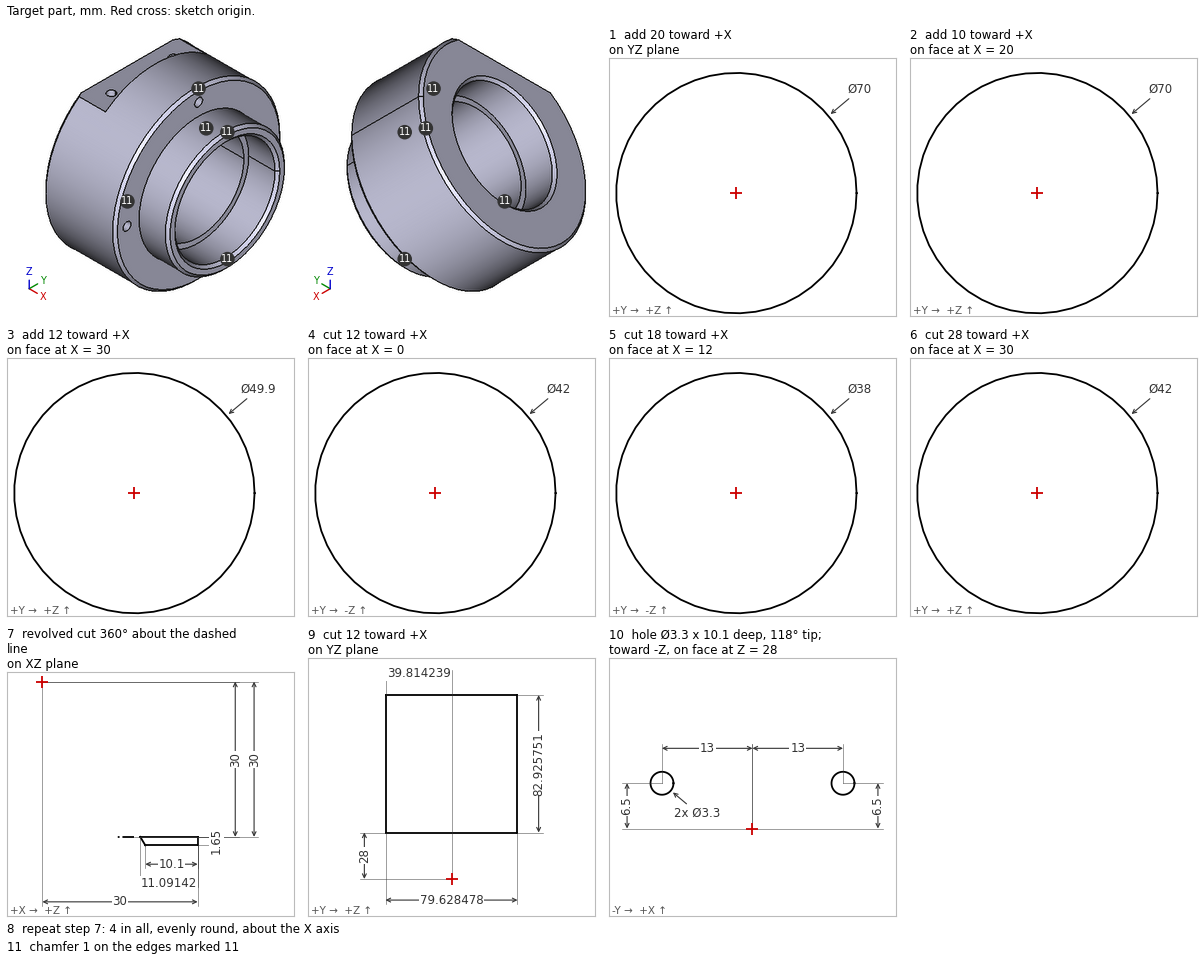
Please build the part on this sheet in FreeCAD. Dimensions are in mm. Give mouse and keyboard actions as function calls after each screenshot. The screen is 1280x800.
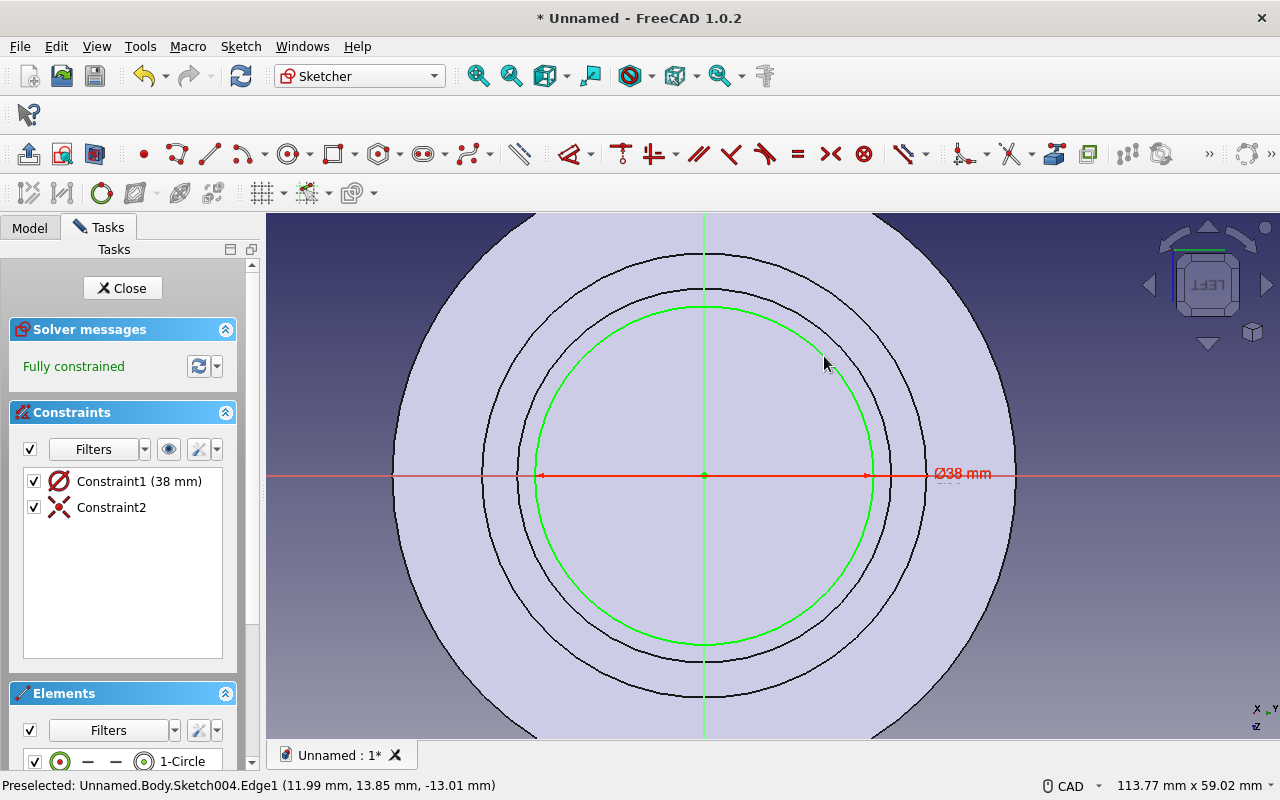
click(123, 288)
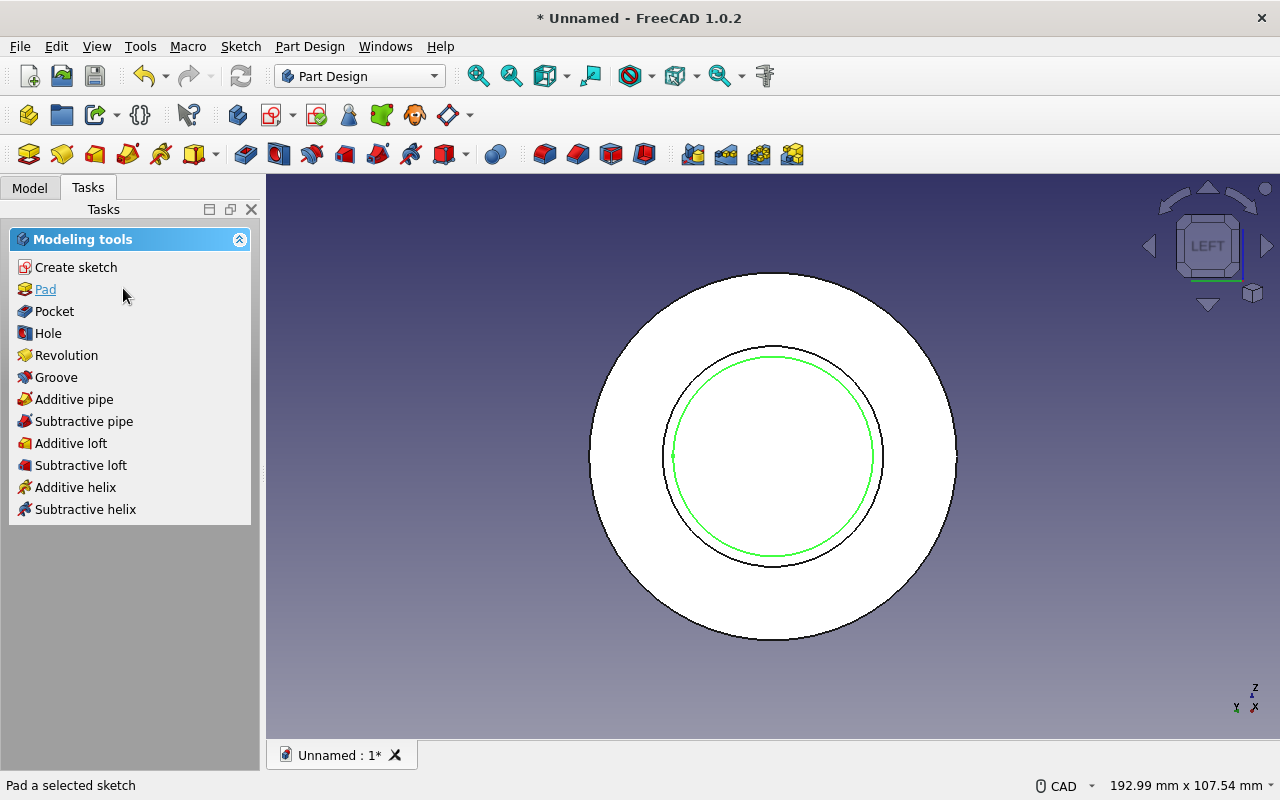
click(246, 154)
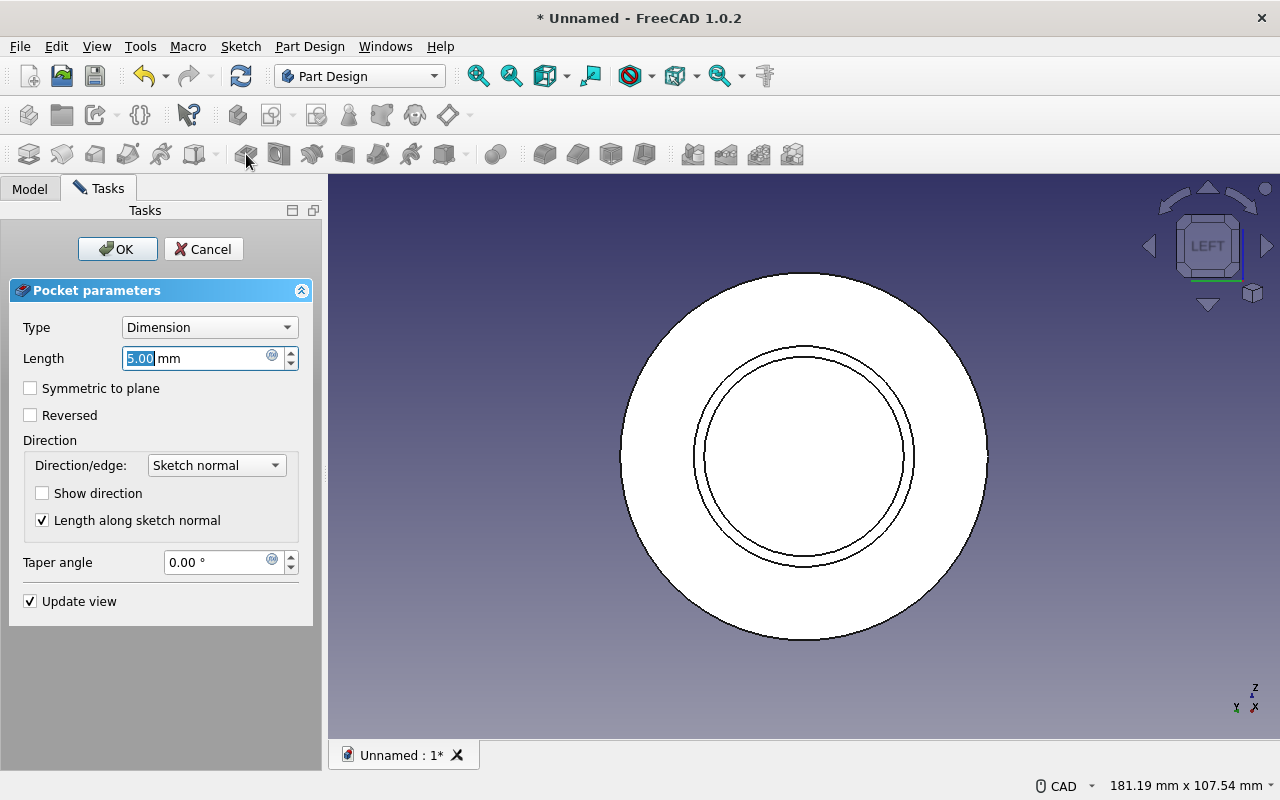
text(18)
key(Tab)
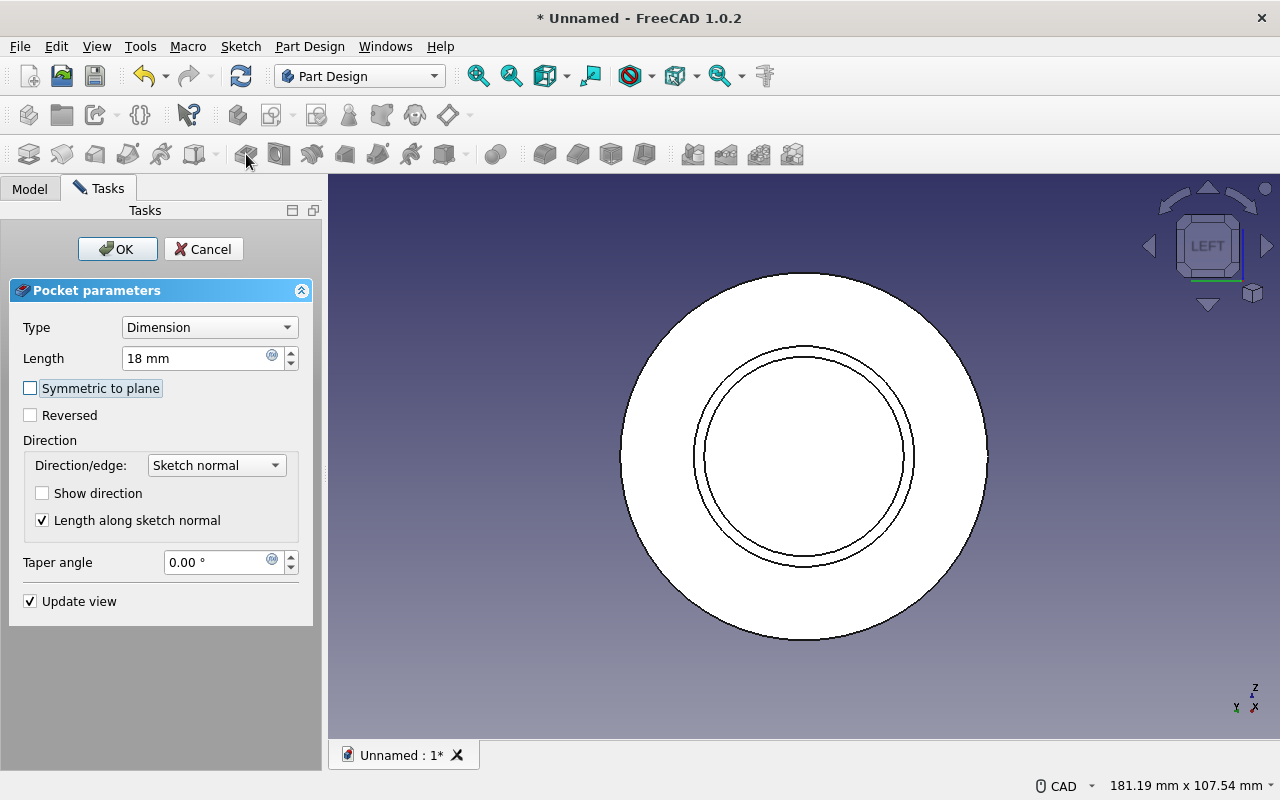
click(118, 249)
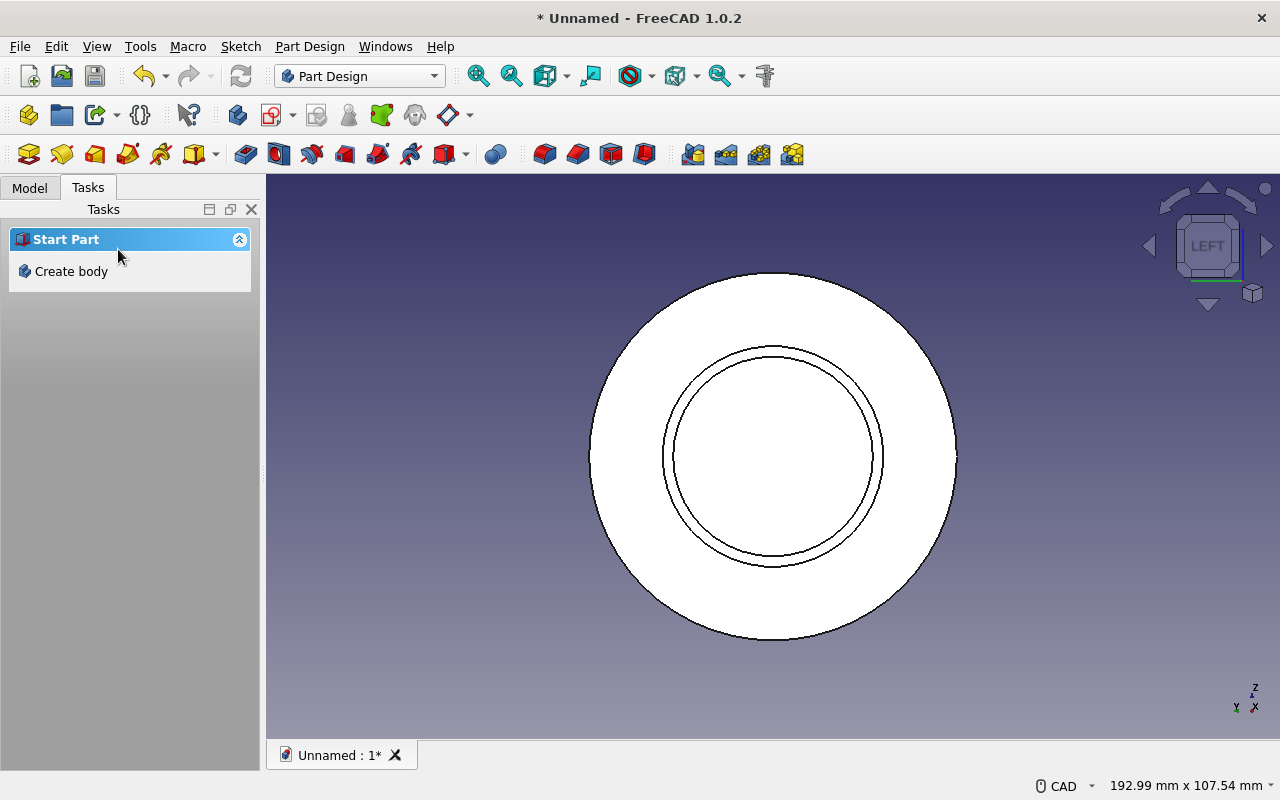
key(0)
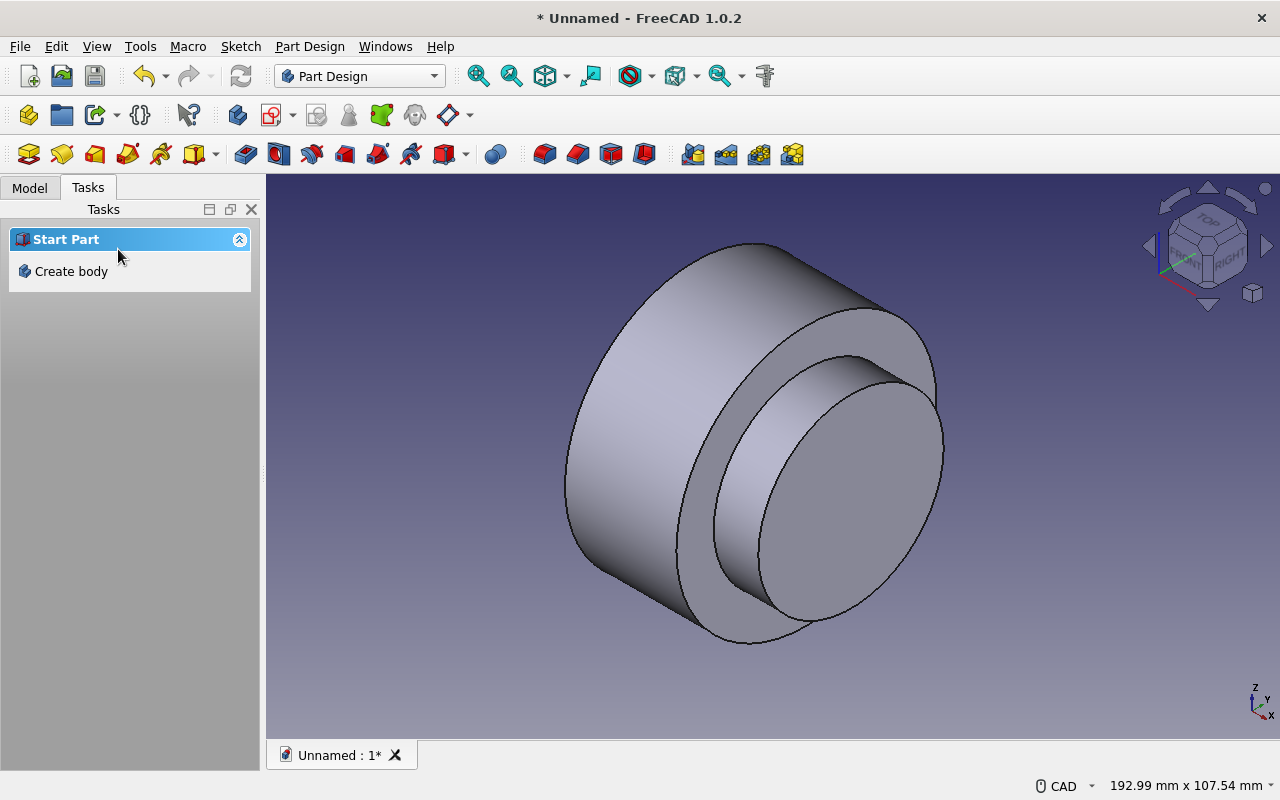
click(806, 346)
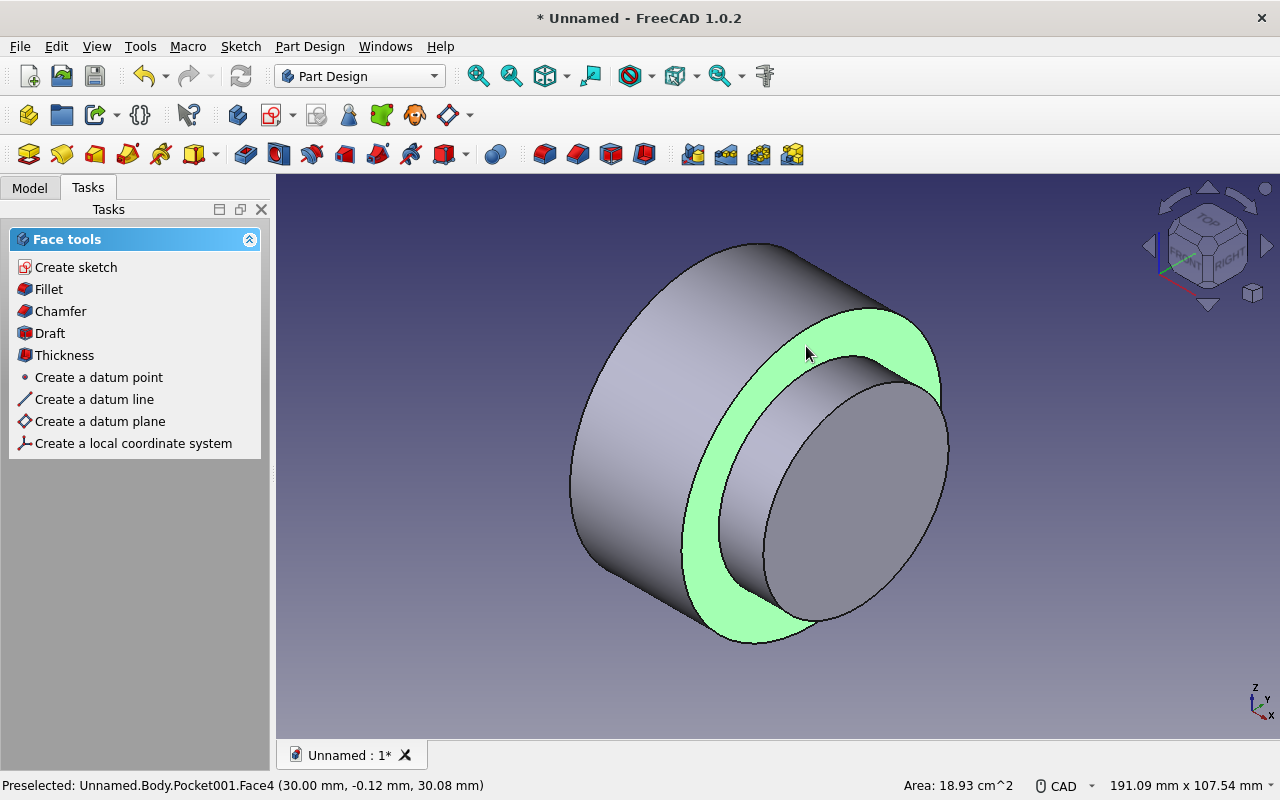
click(270, 116)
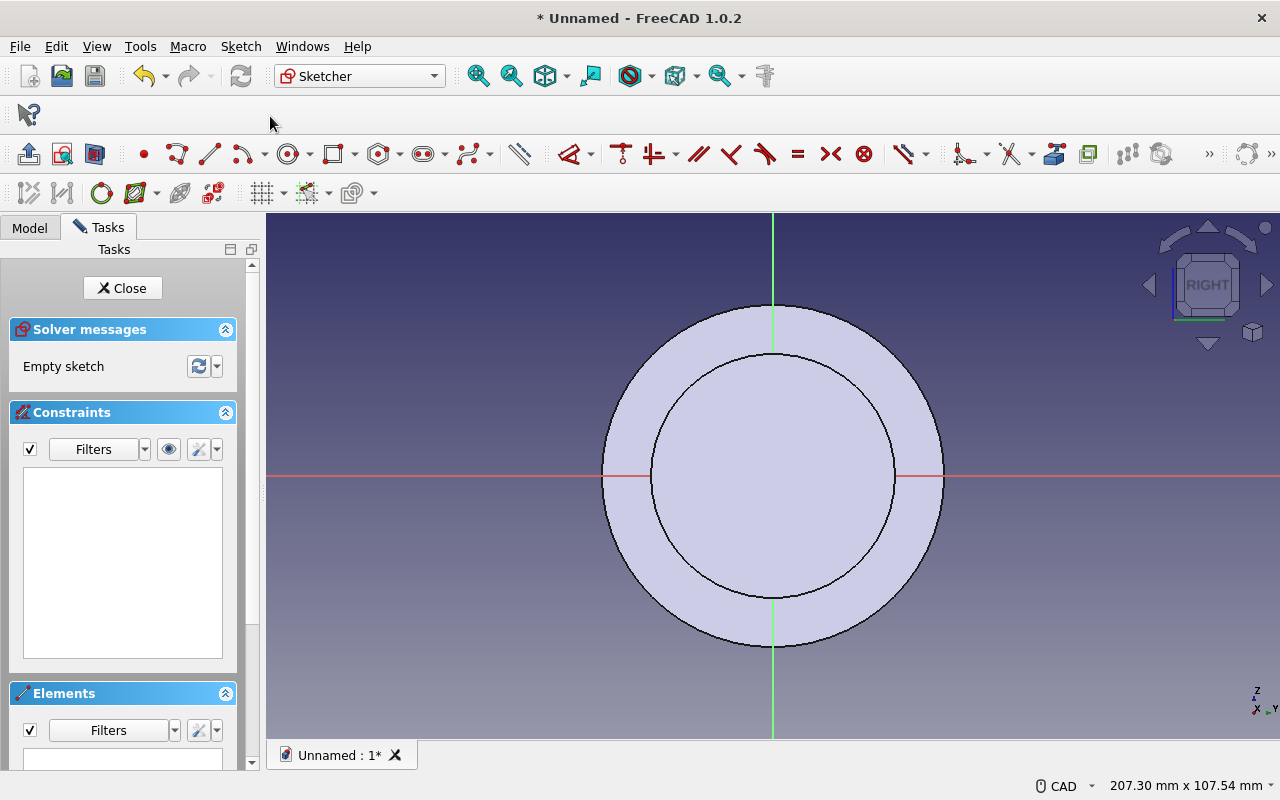
click(95, 154)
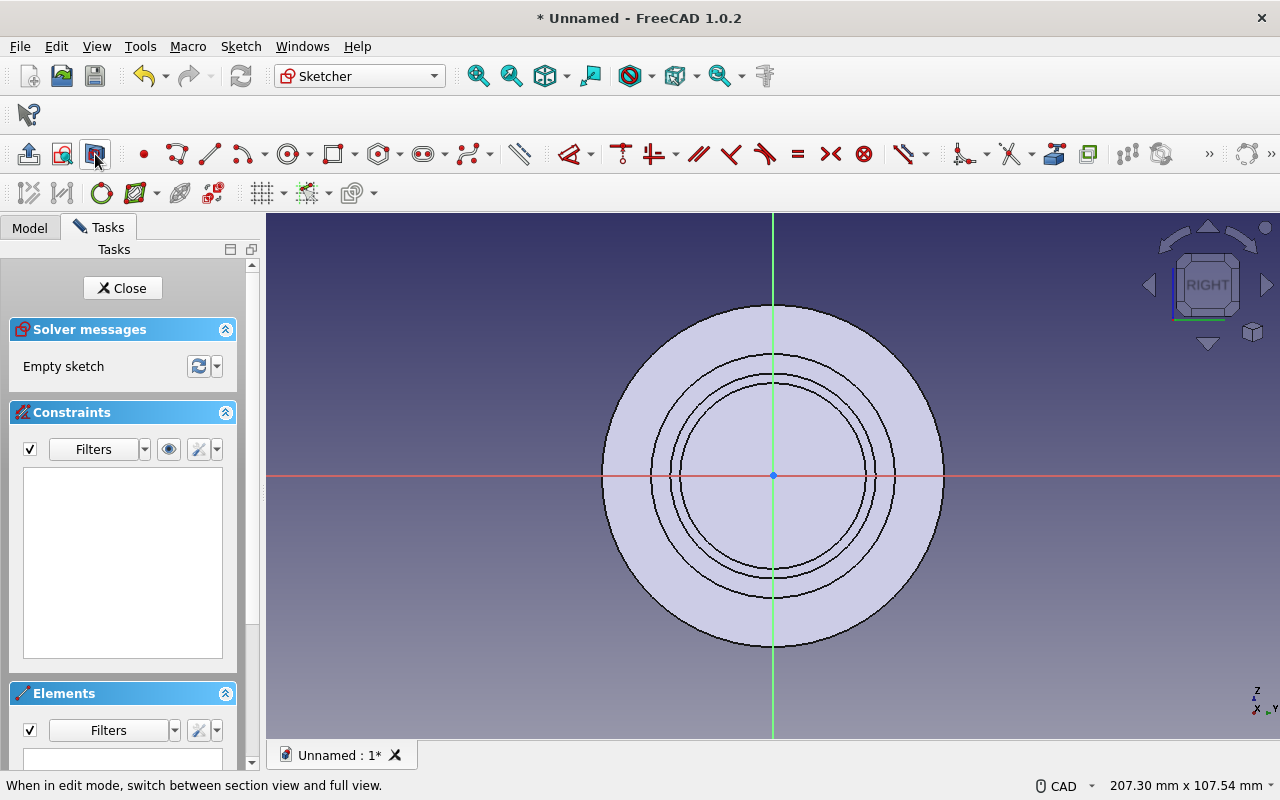
scroll(912, 476, up, 2)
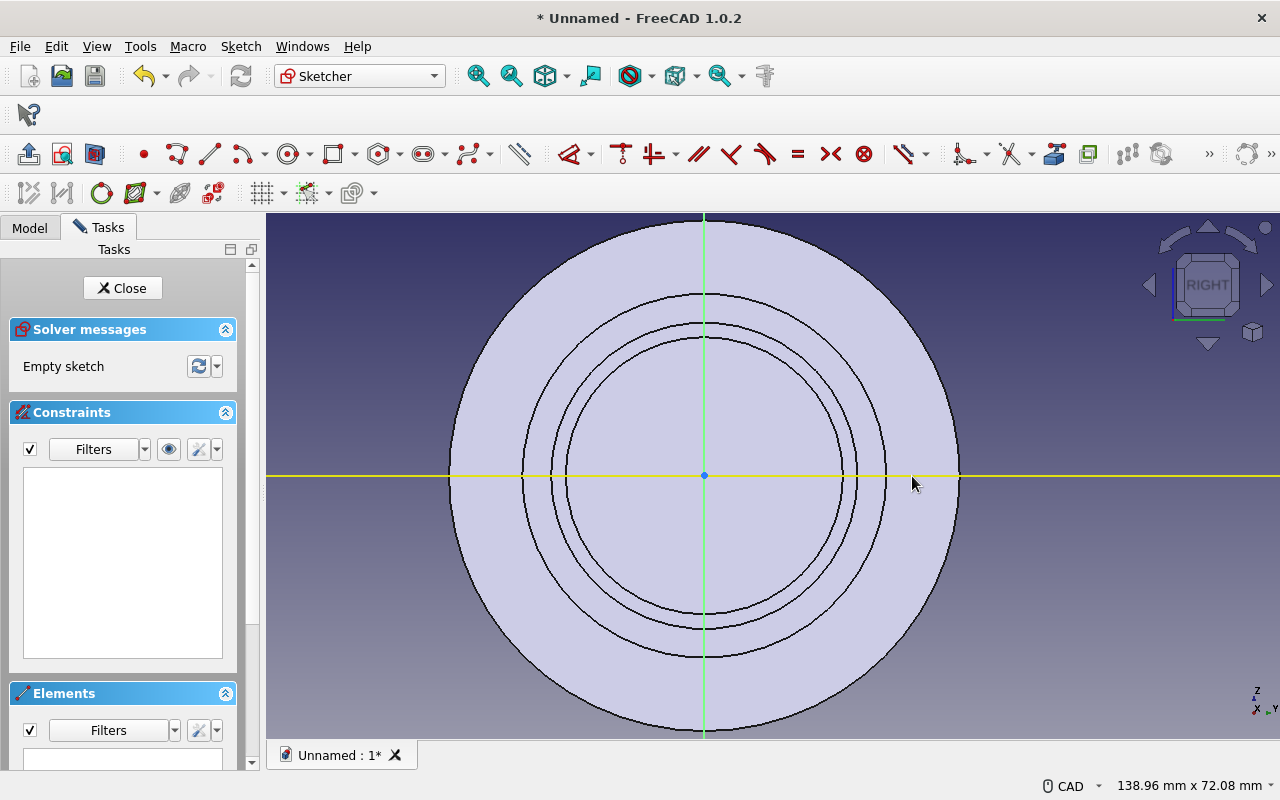
click(288, 154)